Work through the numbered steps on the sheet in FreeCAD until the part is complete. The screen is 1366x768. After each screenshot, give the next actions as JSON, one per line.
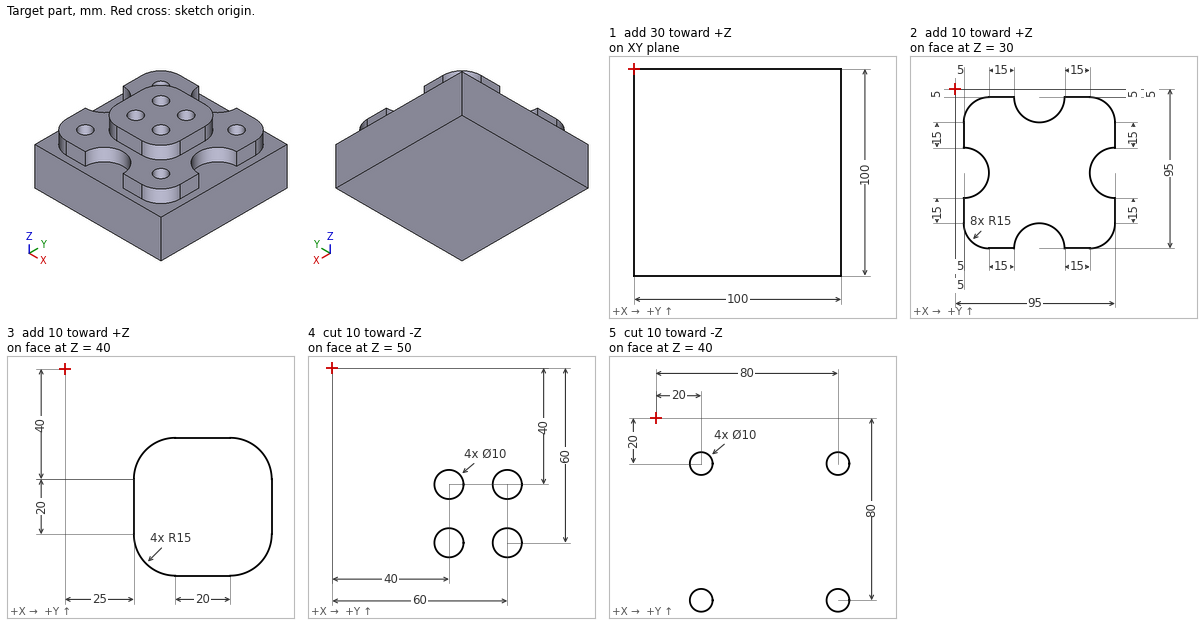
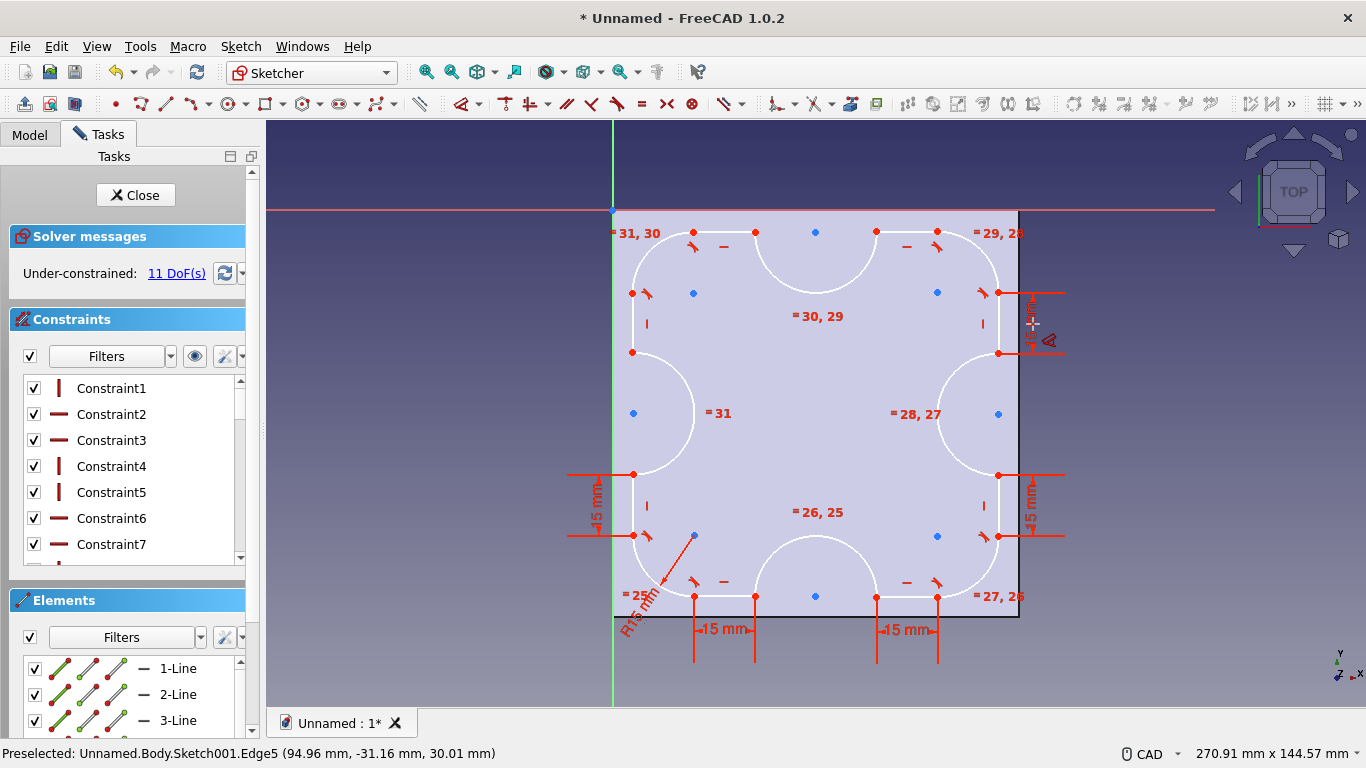
{"action": "left_click", "coordinate": [919, 232]}
{"action": "left_click", "coordinate": [907, 266]}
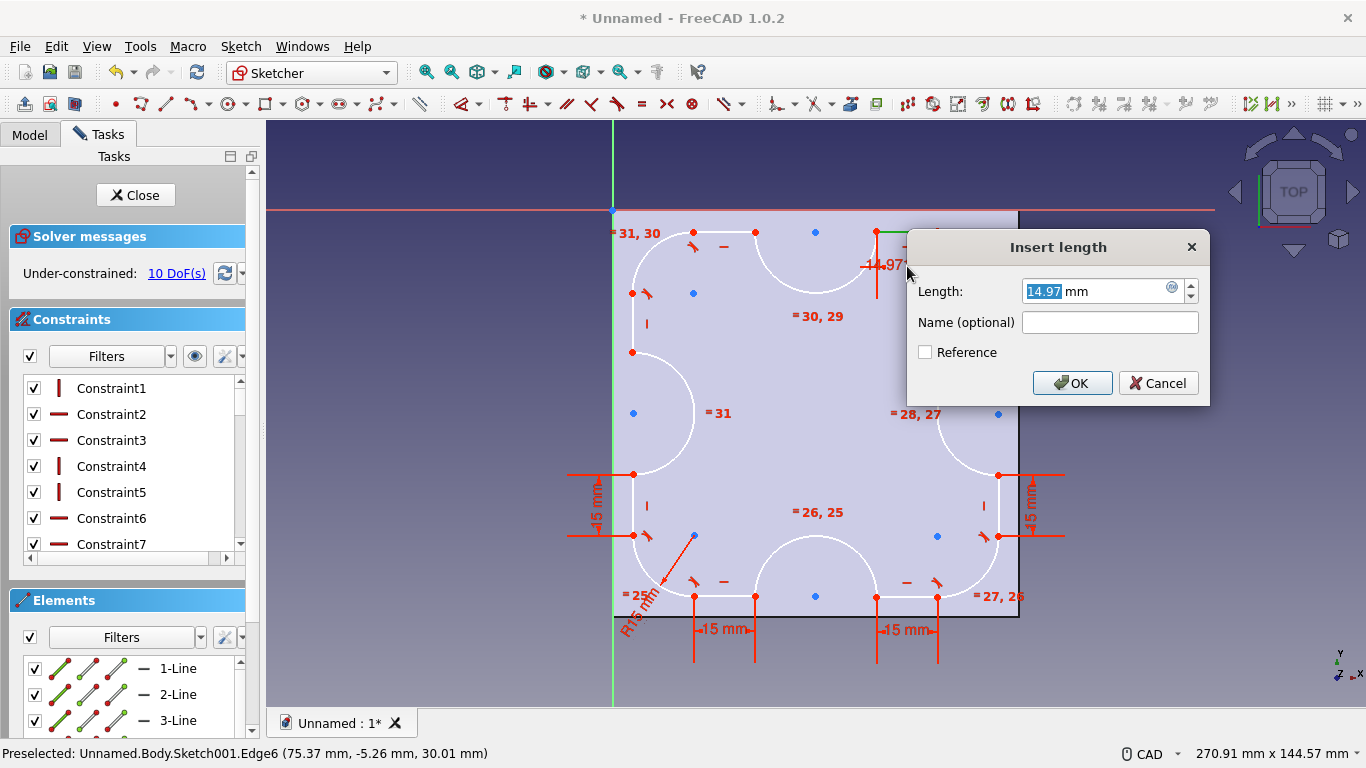
{"action": "type", "text": "15"}
{"action": "key", "text": "Return"}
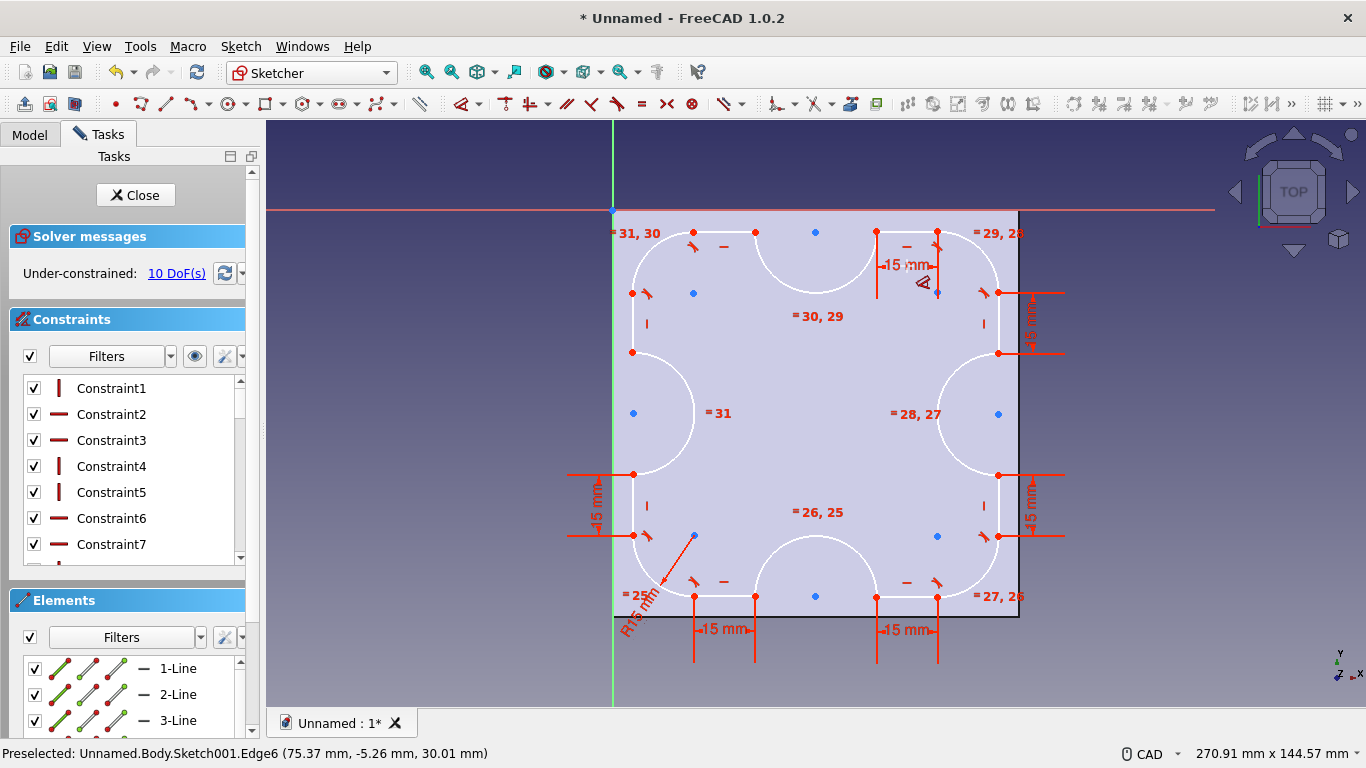
{"action": "left_click", "coordinate": [737, 232]}
{"action": "left_click", "coordinate": [724, 266]}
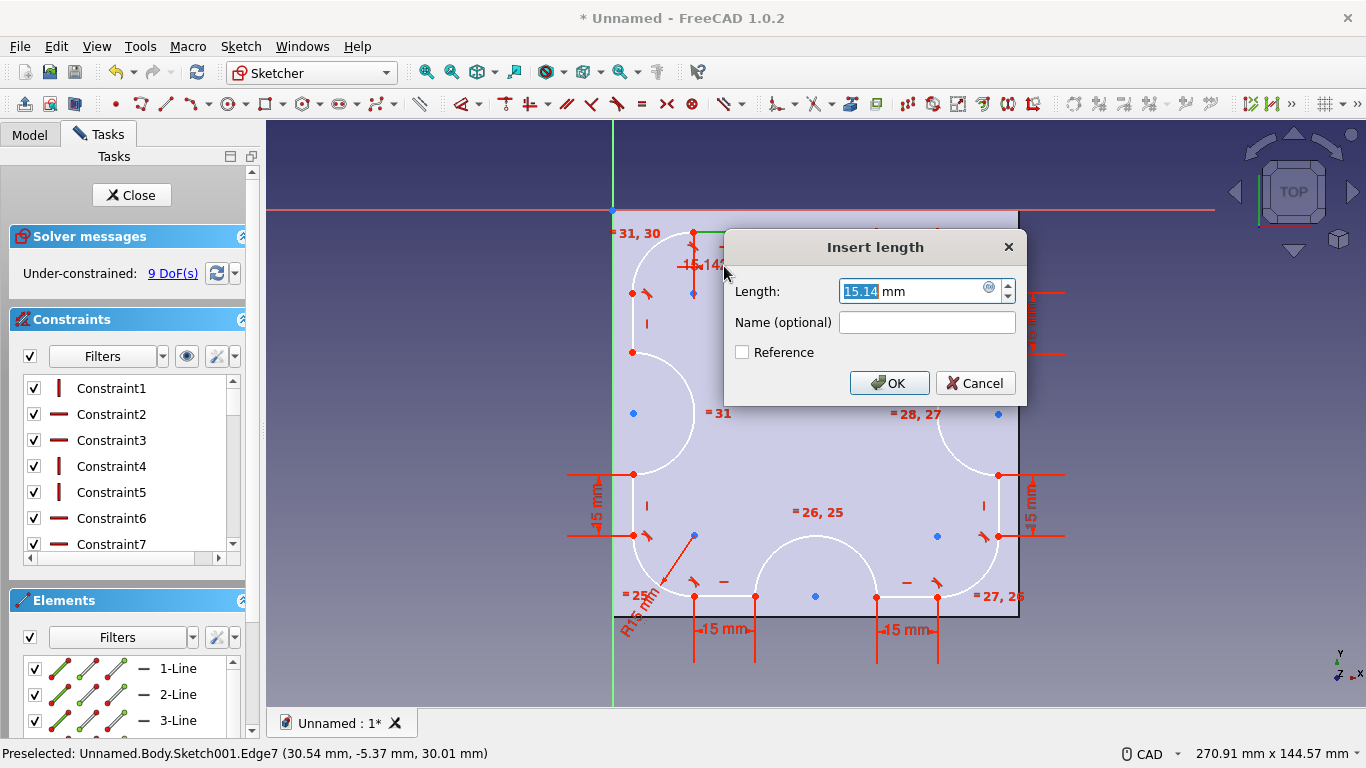
{"action": "type", "text": "15"}
{"action": "key", "text": "Return"}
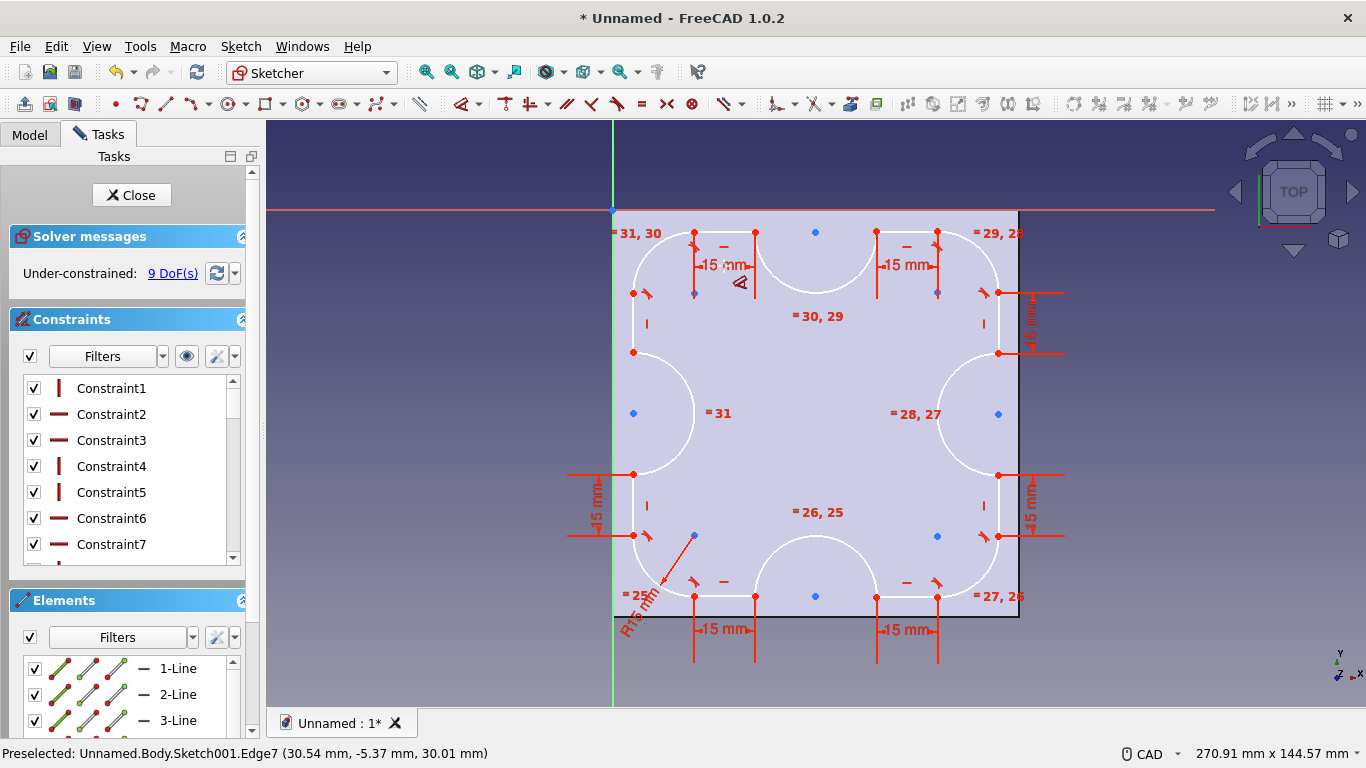
{"action": "left_click", "coordinate": [633, 311]}
{"action": "left_click", "coordinate": [599, 323]}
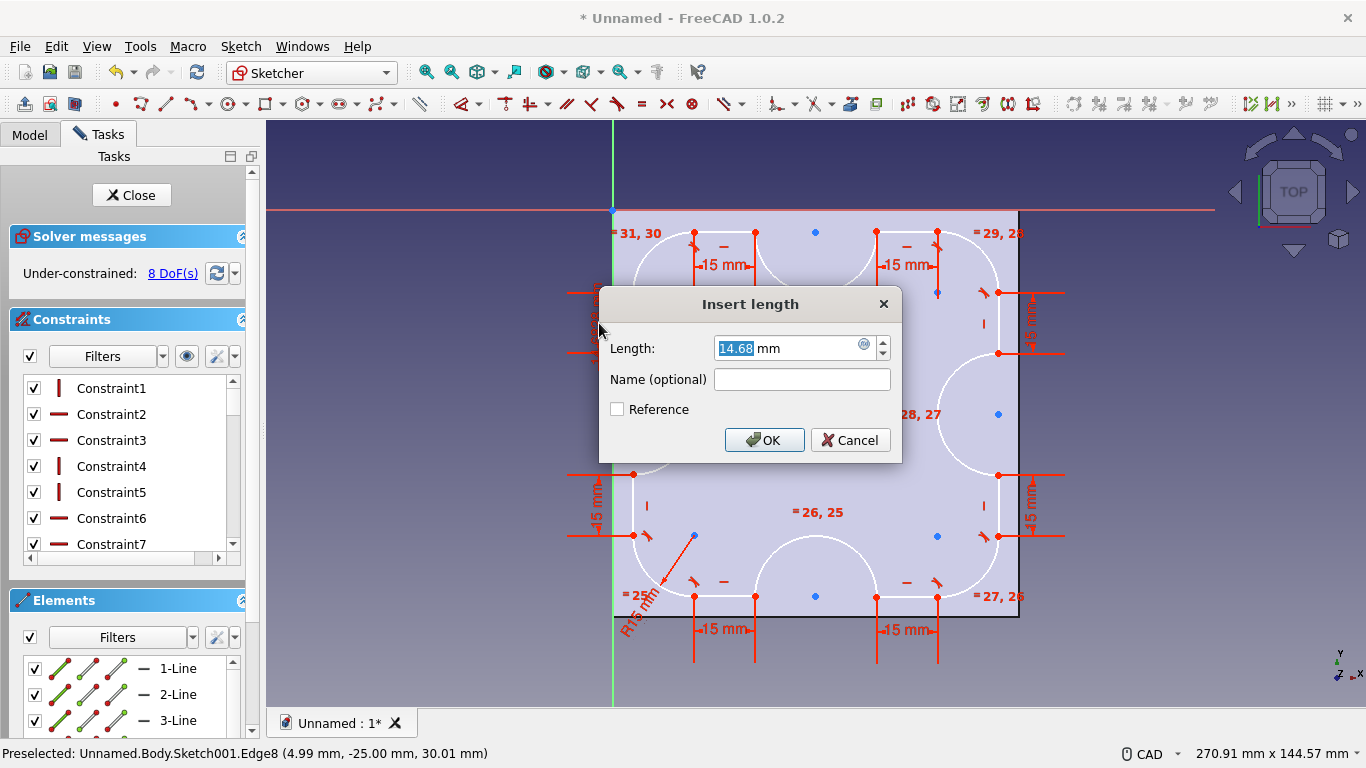
{"action": "type", "text": "15"}
{"action": "key", "text": "Return"}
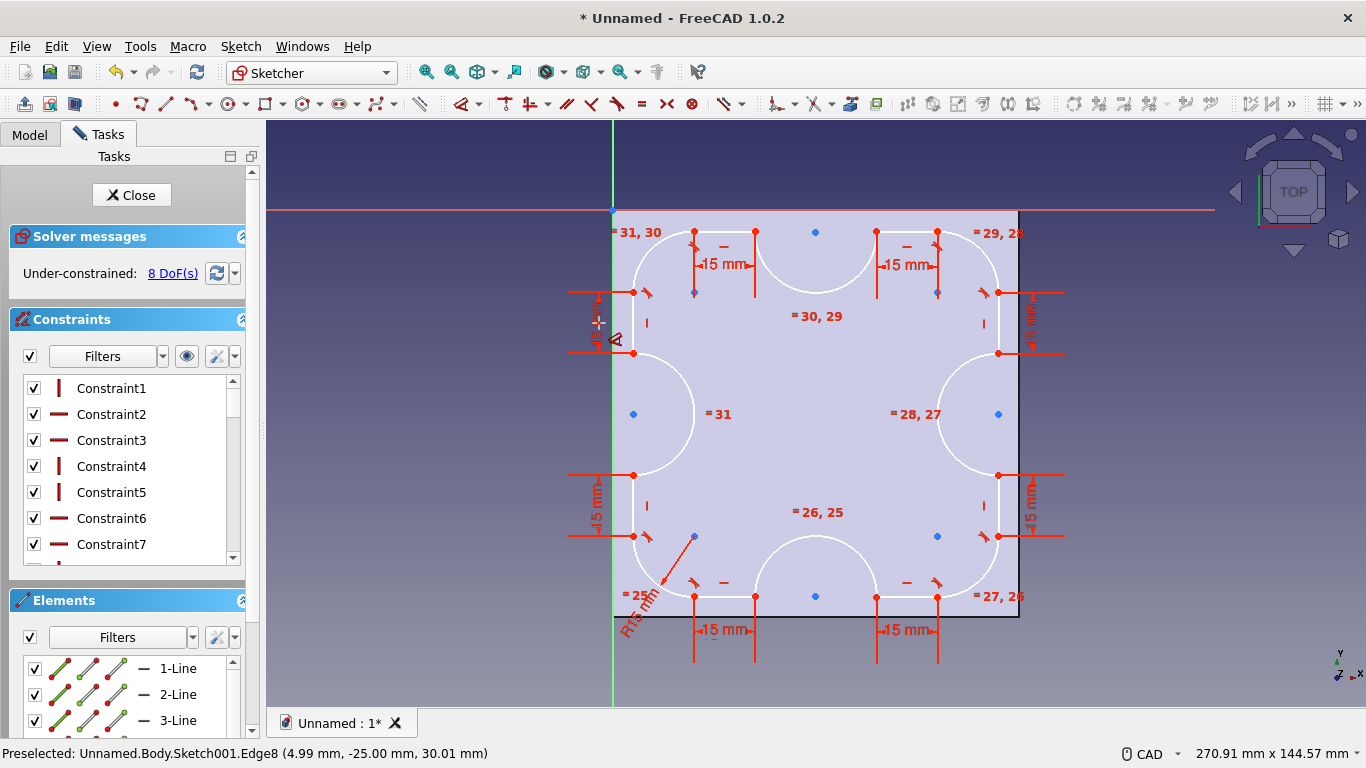
{"action": "scroll", "coordinate": [633, 475], "scroll_direction": "up", "scroll_amount": 4}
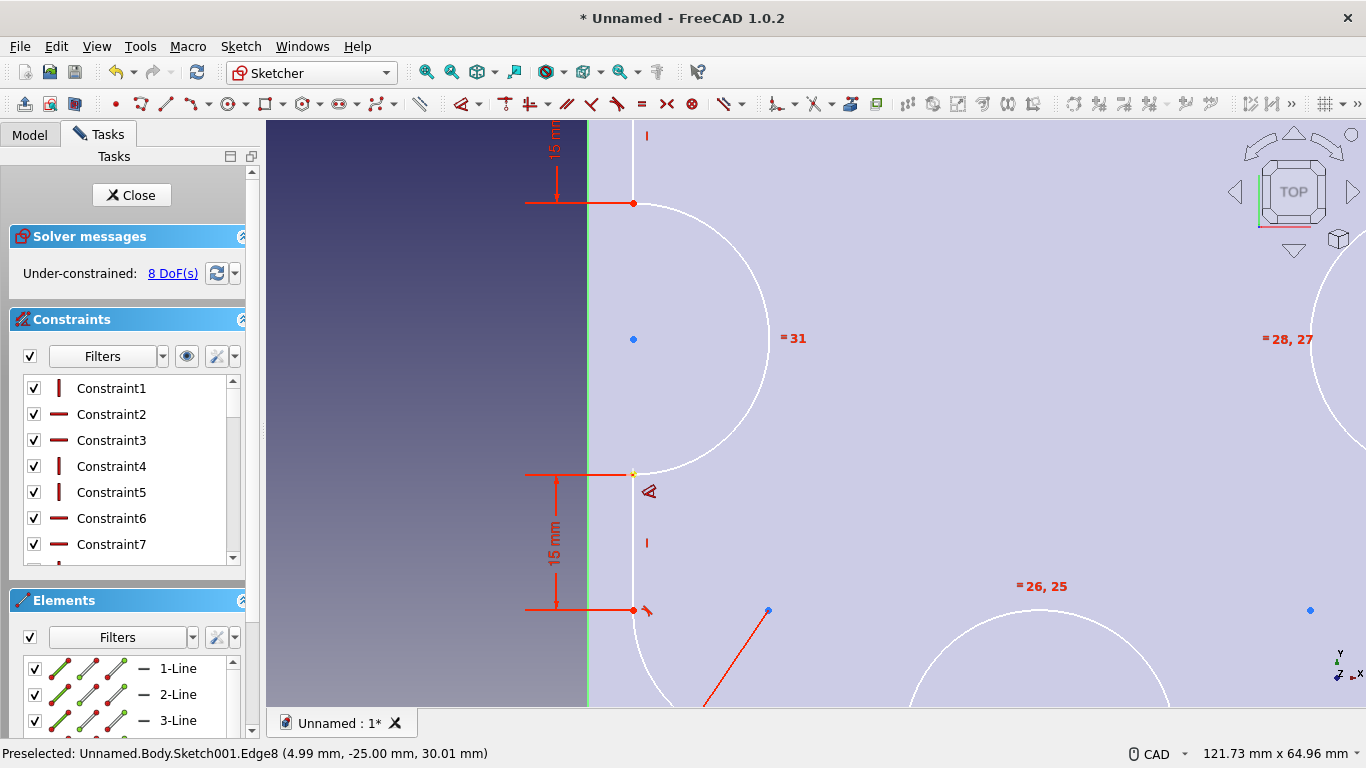
{"action": "left_click", "coordinate": [633, 475]}
{"action": "left_click", "coordinate": [611, 509]}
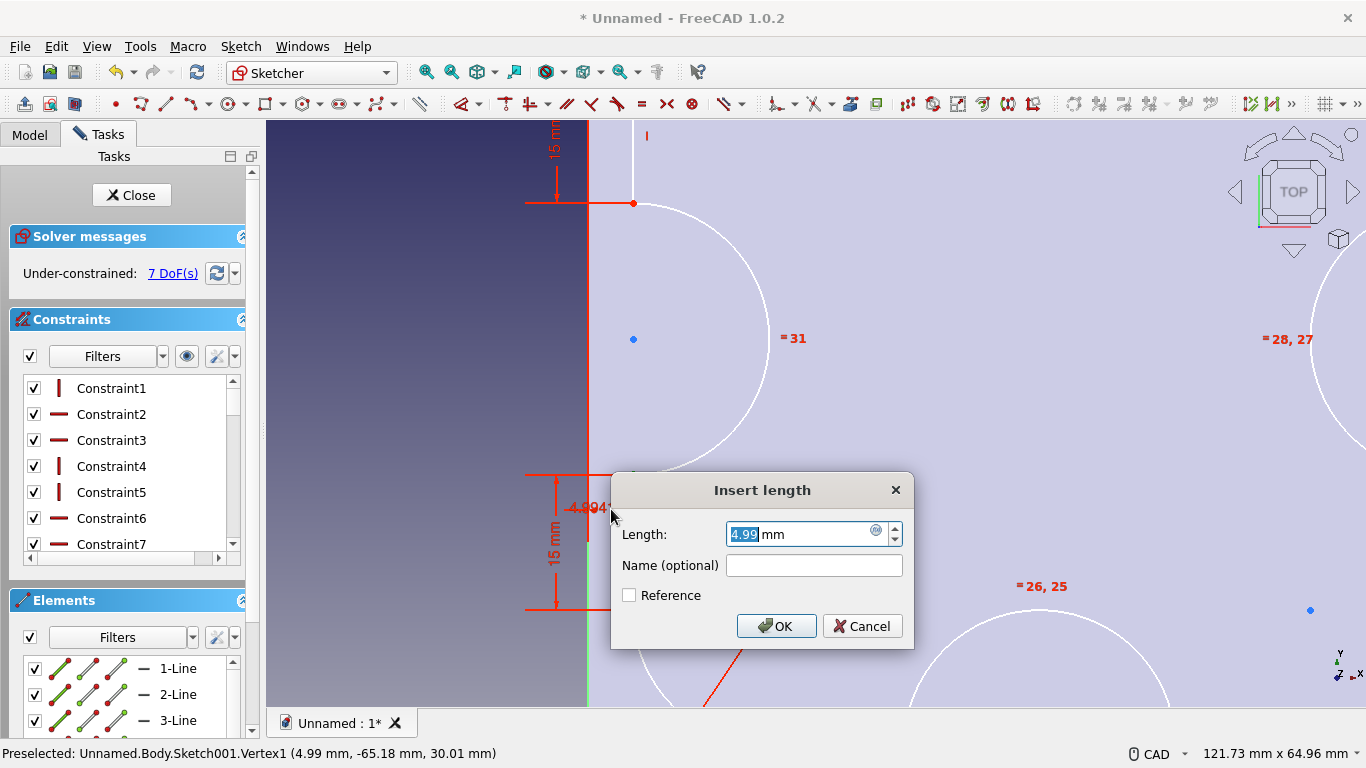
{"action": "type", "text": "5"}
{"action": "key", "text": "Return"}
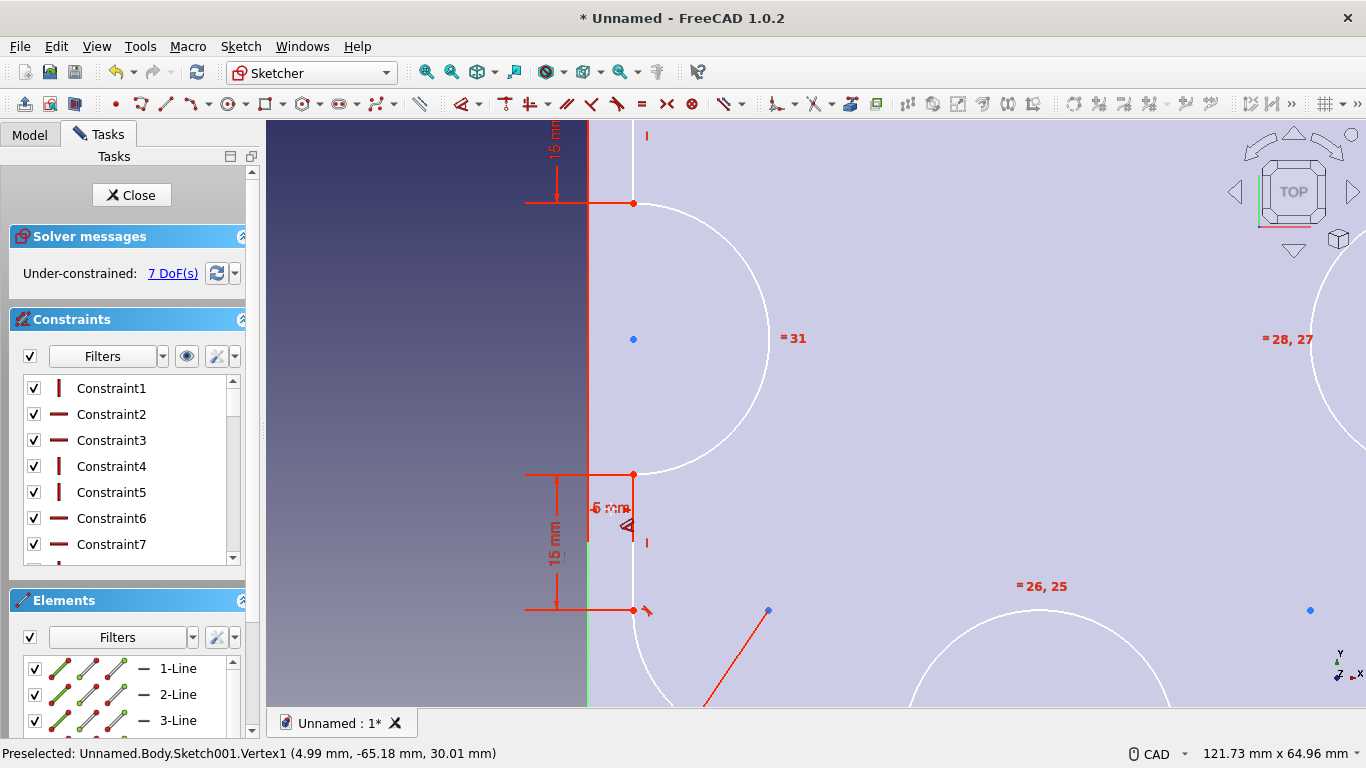
{"action": "scroll", "coordinate": [527, 494], "scroll_direction": "down", "scroll_amount": 4}